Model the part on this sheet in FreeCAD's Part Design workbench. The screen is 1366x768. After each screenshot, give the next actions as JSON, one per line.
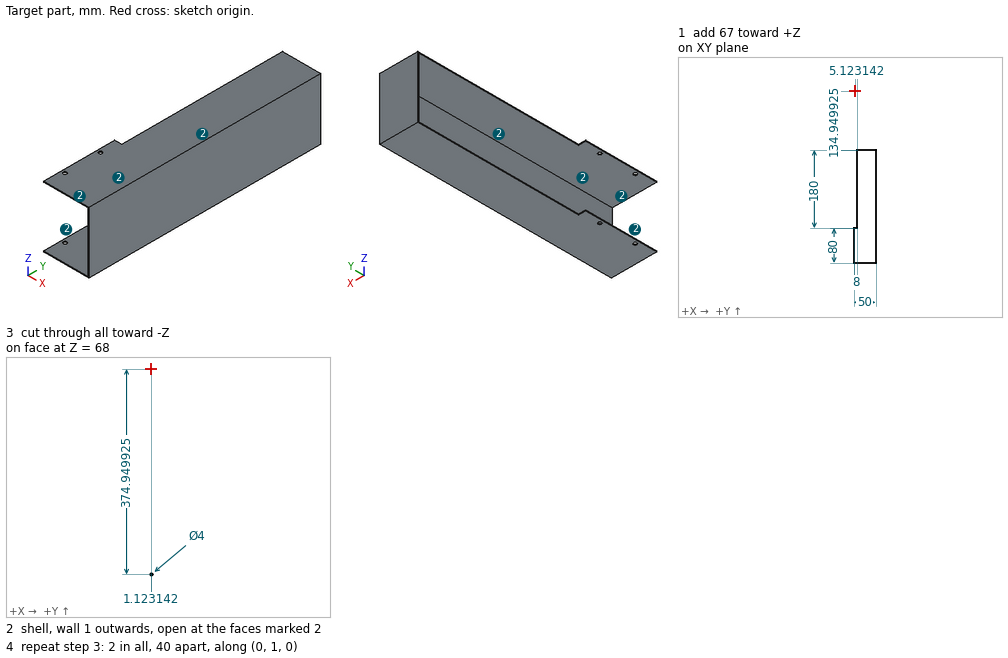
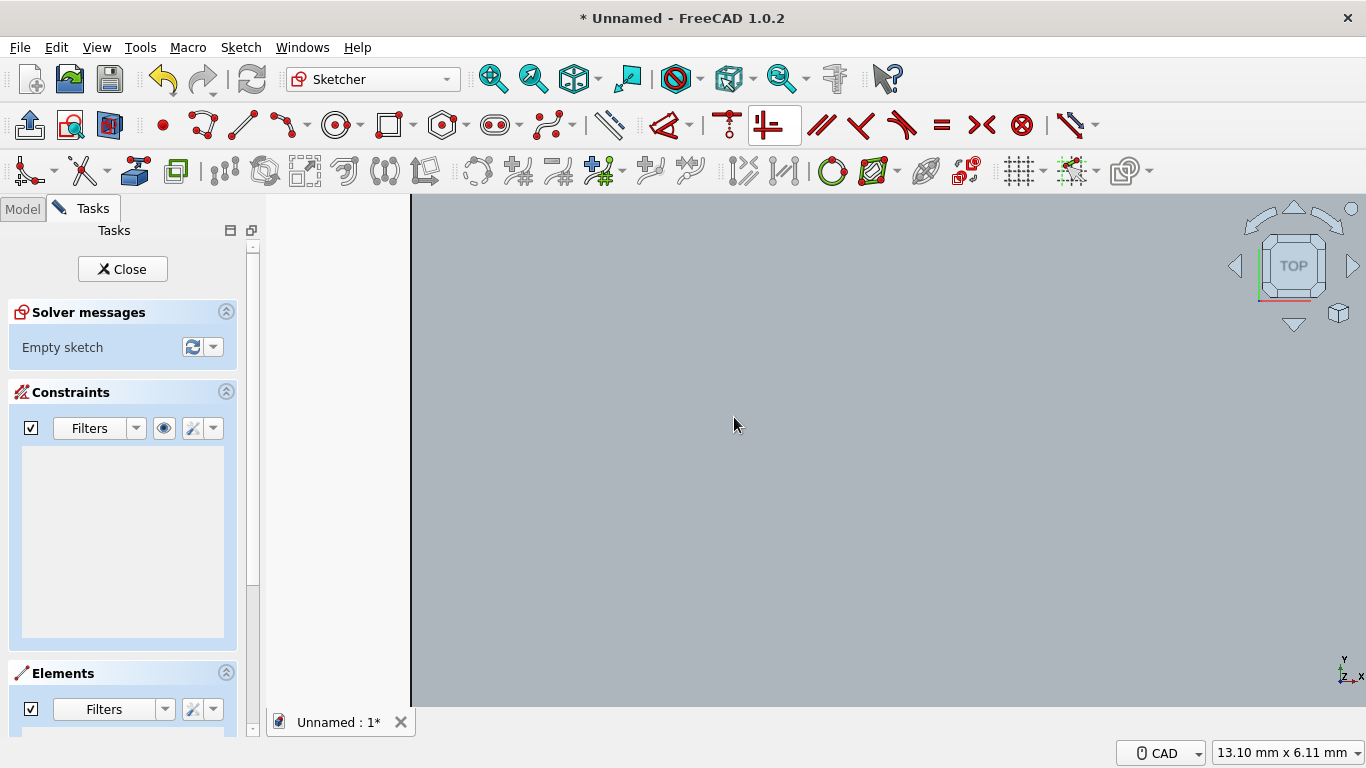
{"action": "left_click", "coordinate": [336, 126]}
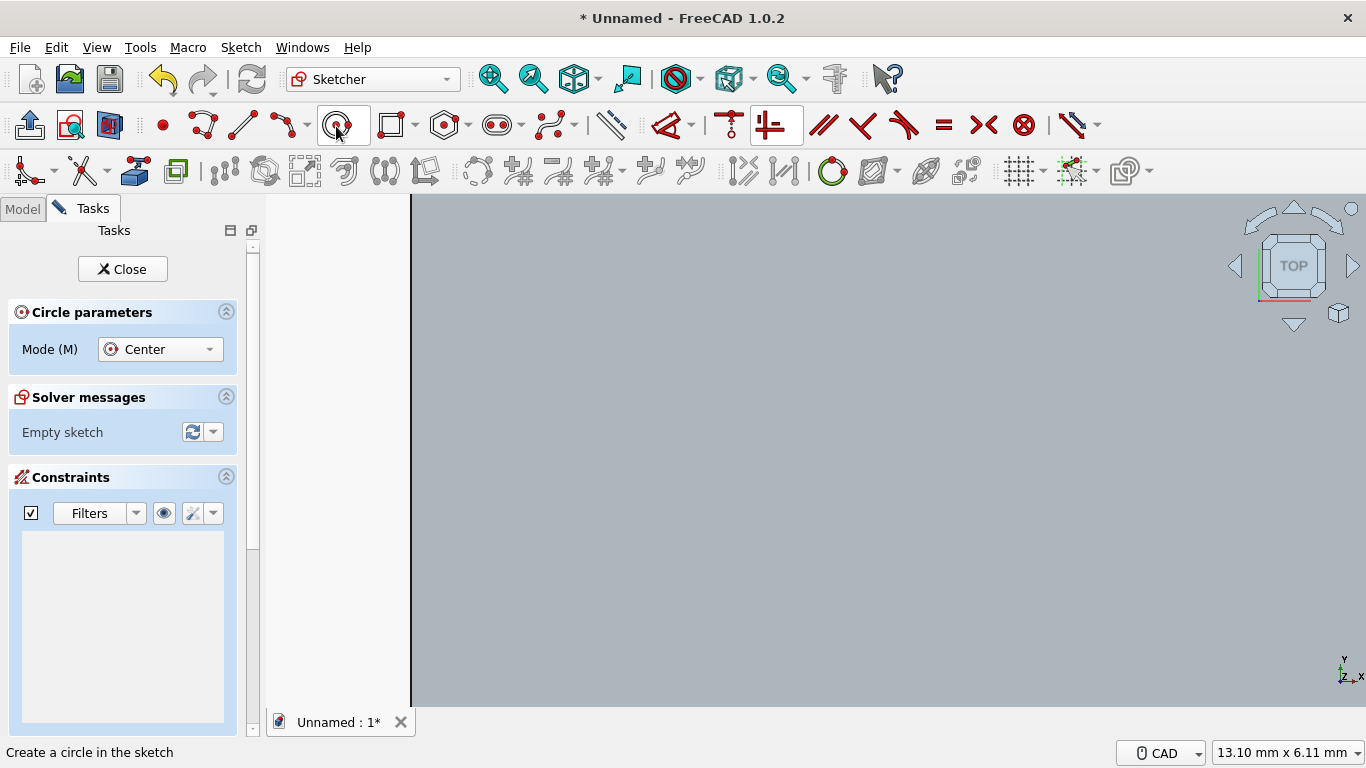
{"action": "left_click", "coordinate": [747, 449]}
{"action": "left_click", "coordinate": [866, 331]}
{"action": "key", "text": "Escape"}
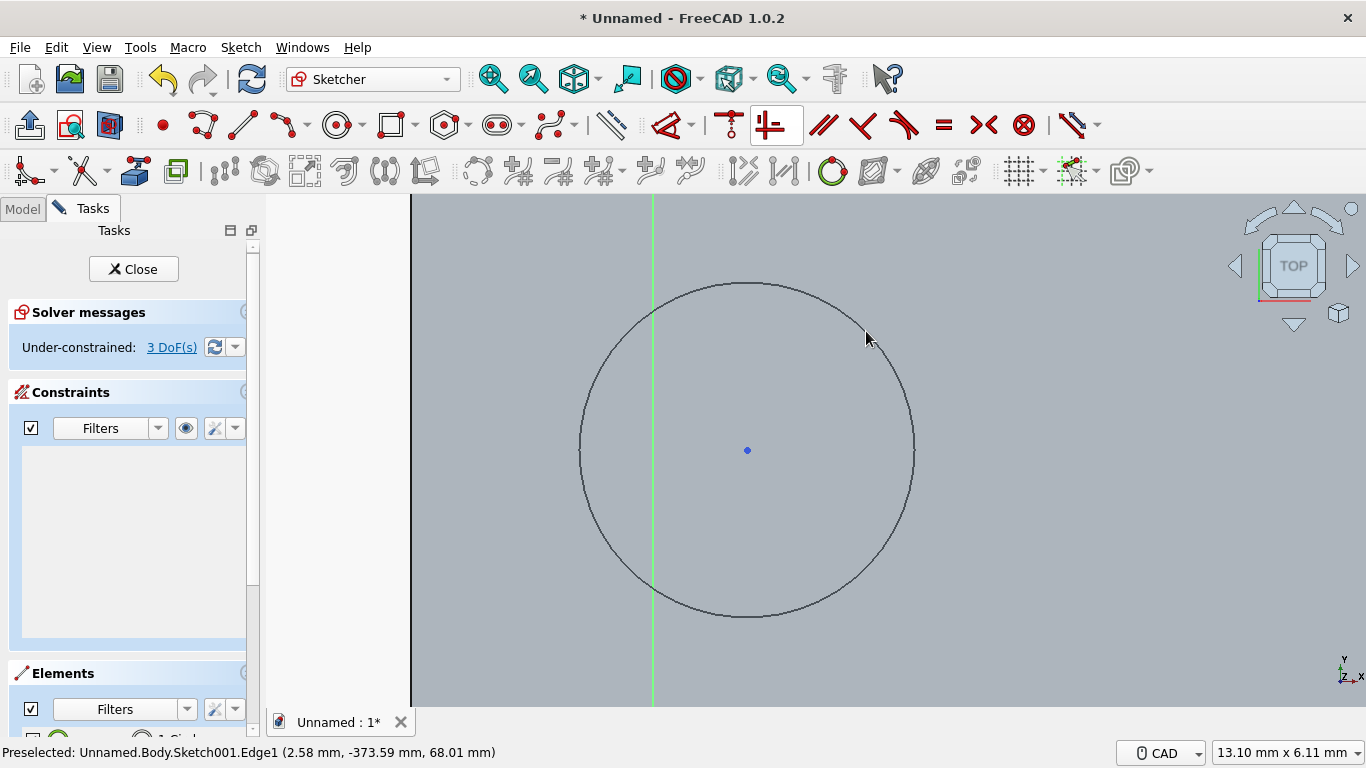
{"action": "left_click", "coordinate": [666, 126]}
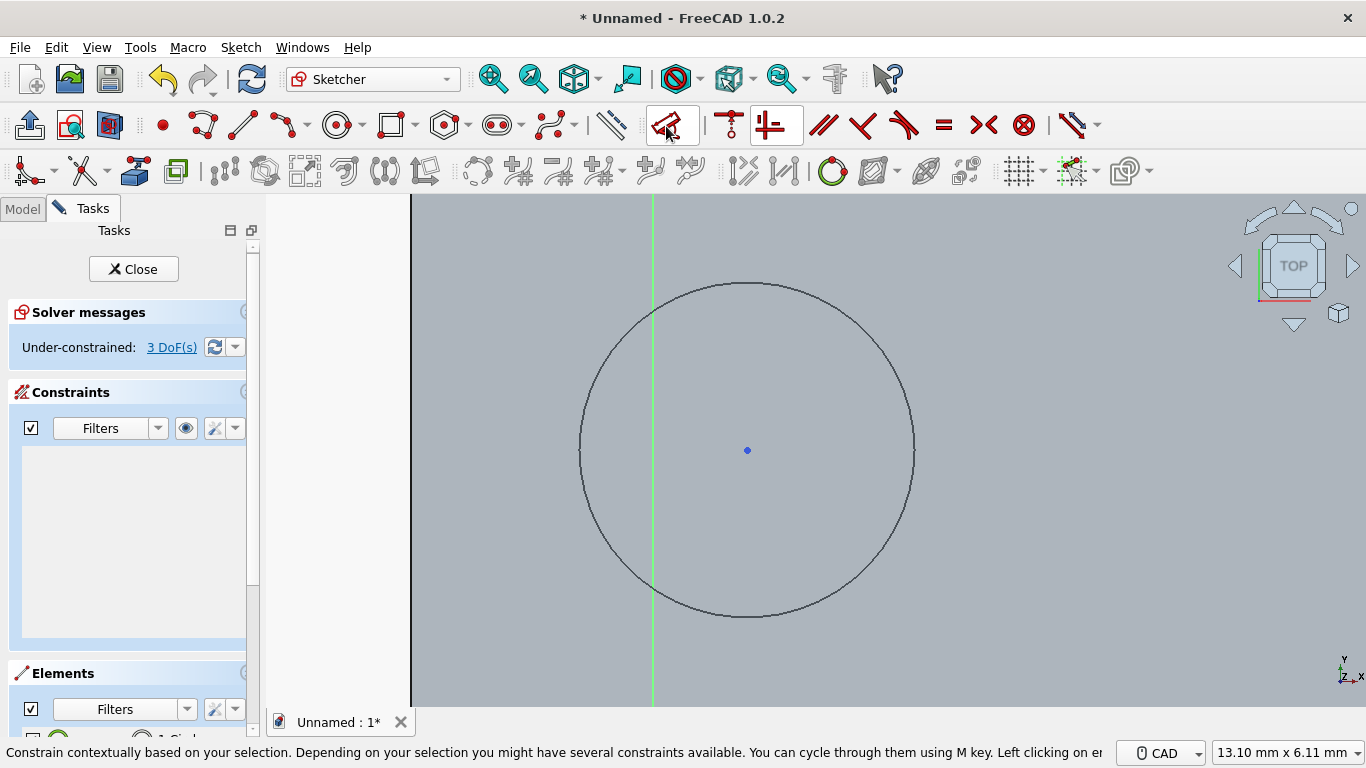
{"action": "left_click", "coordinate": [865, 331]}
{"action": "left_click", "coordinate": [888, 308]}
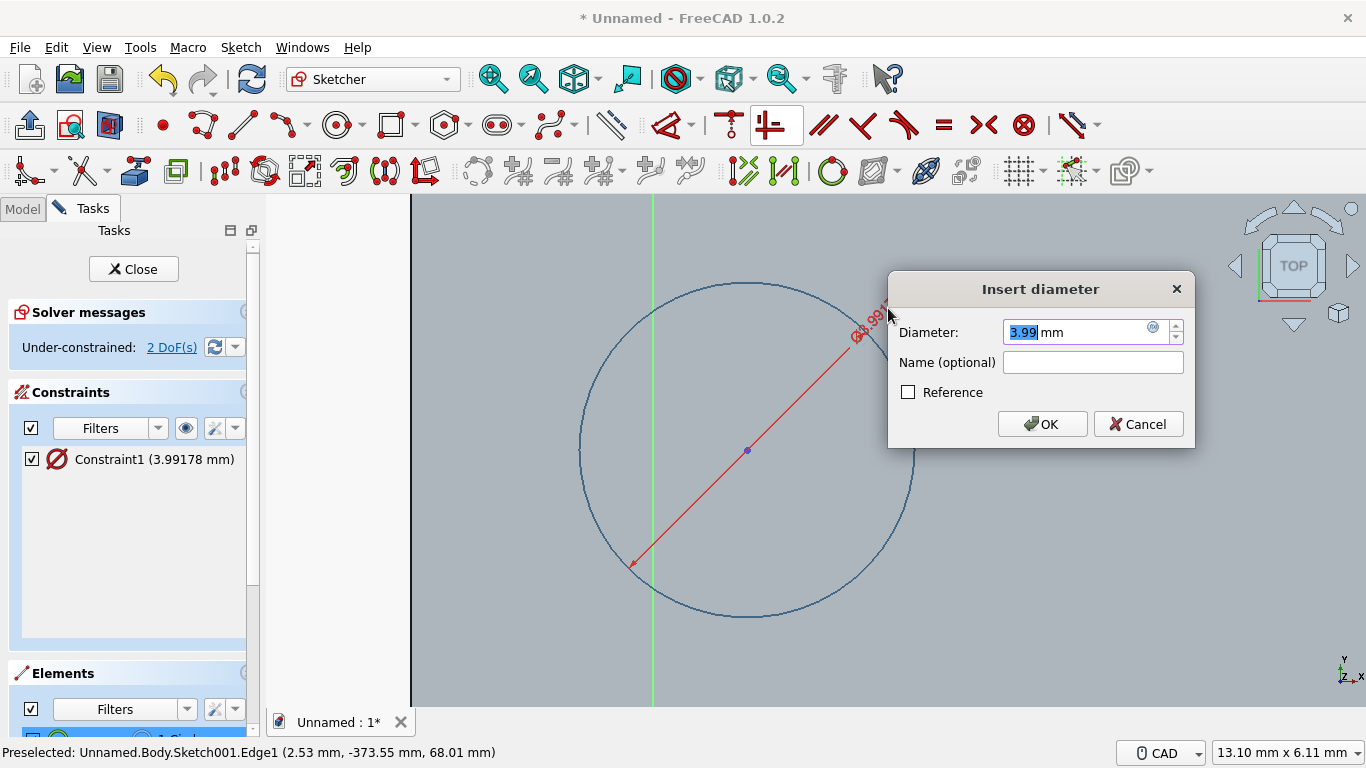
{"action": "type", "text": "4"}
{"action": "key", "text": "Return"}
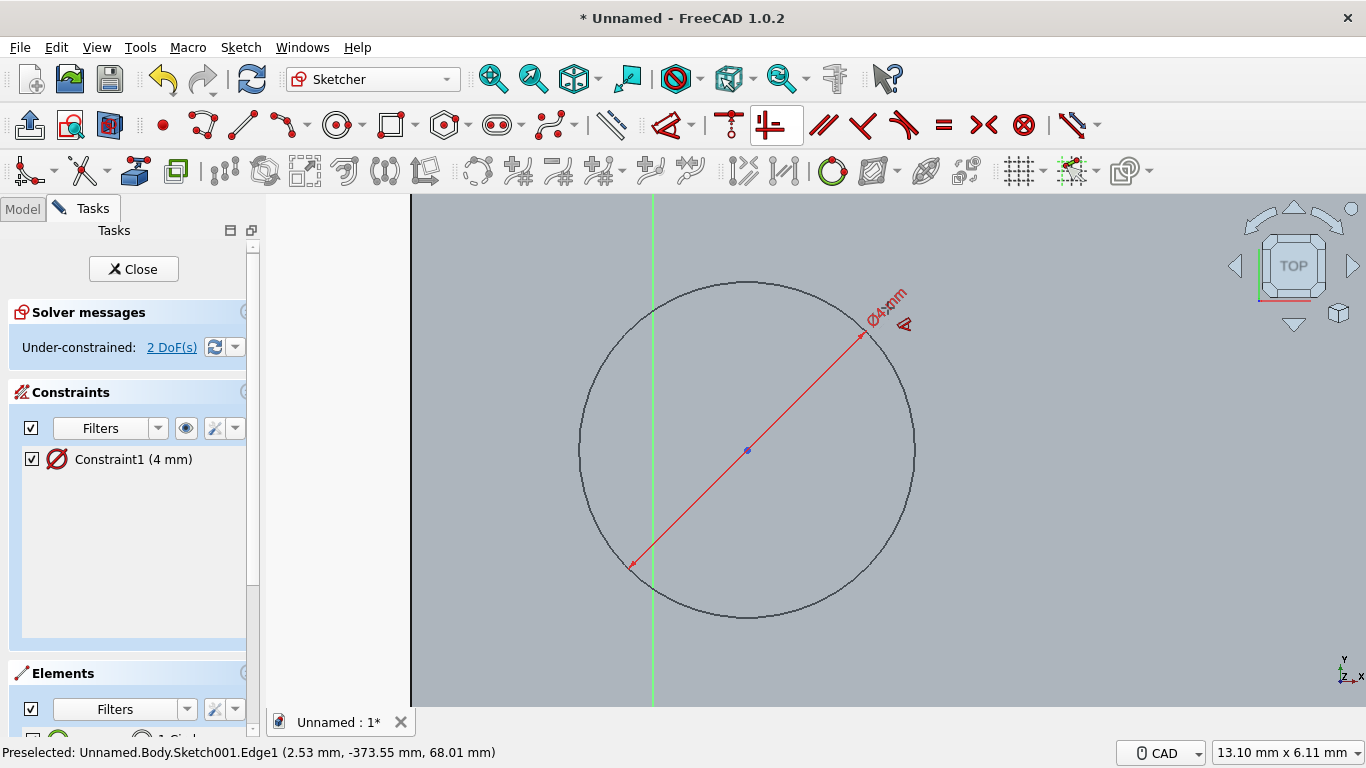
{"action": "left_click", "coordinate": [747, 450]}
{"action": "left_click", "coordinate": [700, 484]}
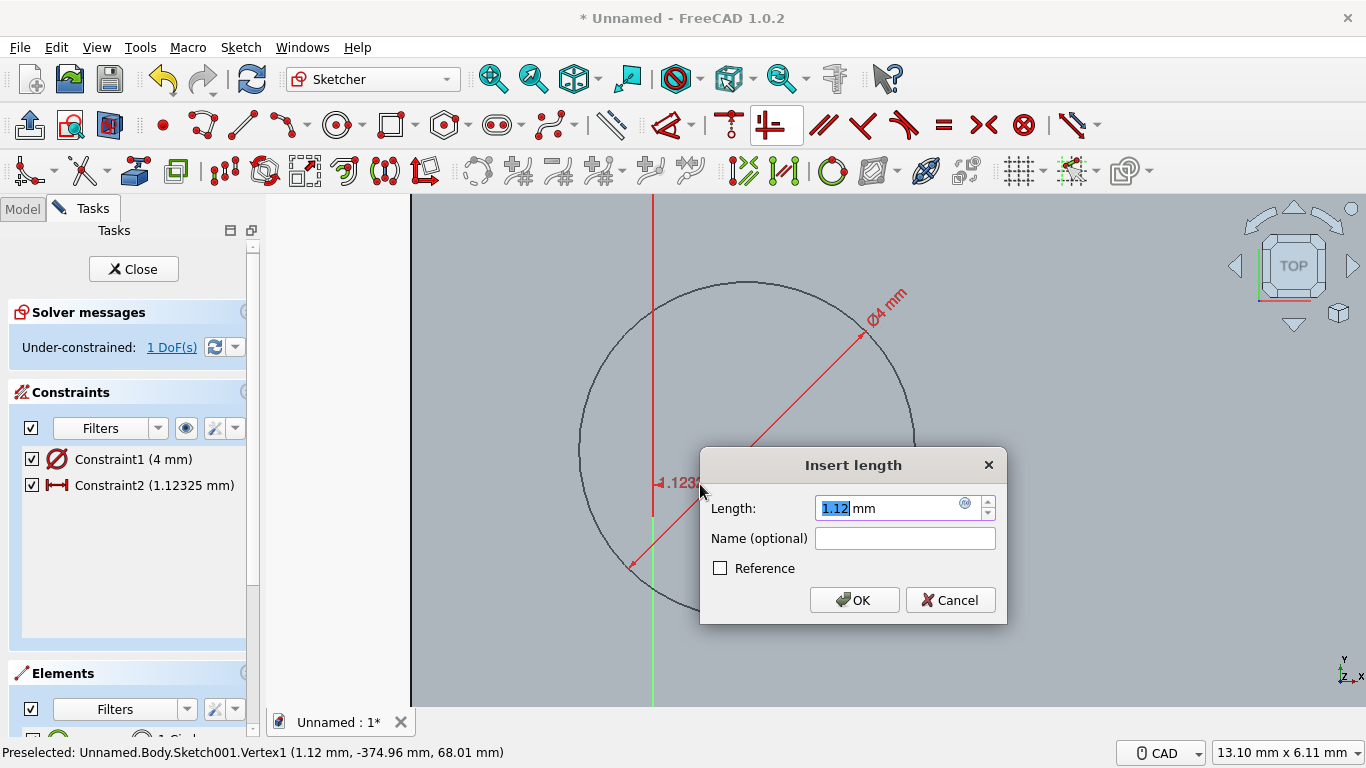
{"action": "type", "text": "1.123142"}
{"action": "key", "text": "Return"}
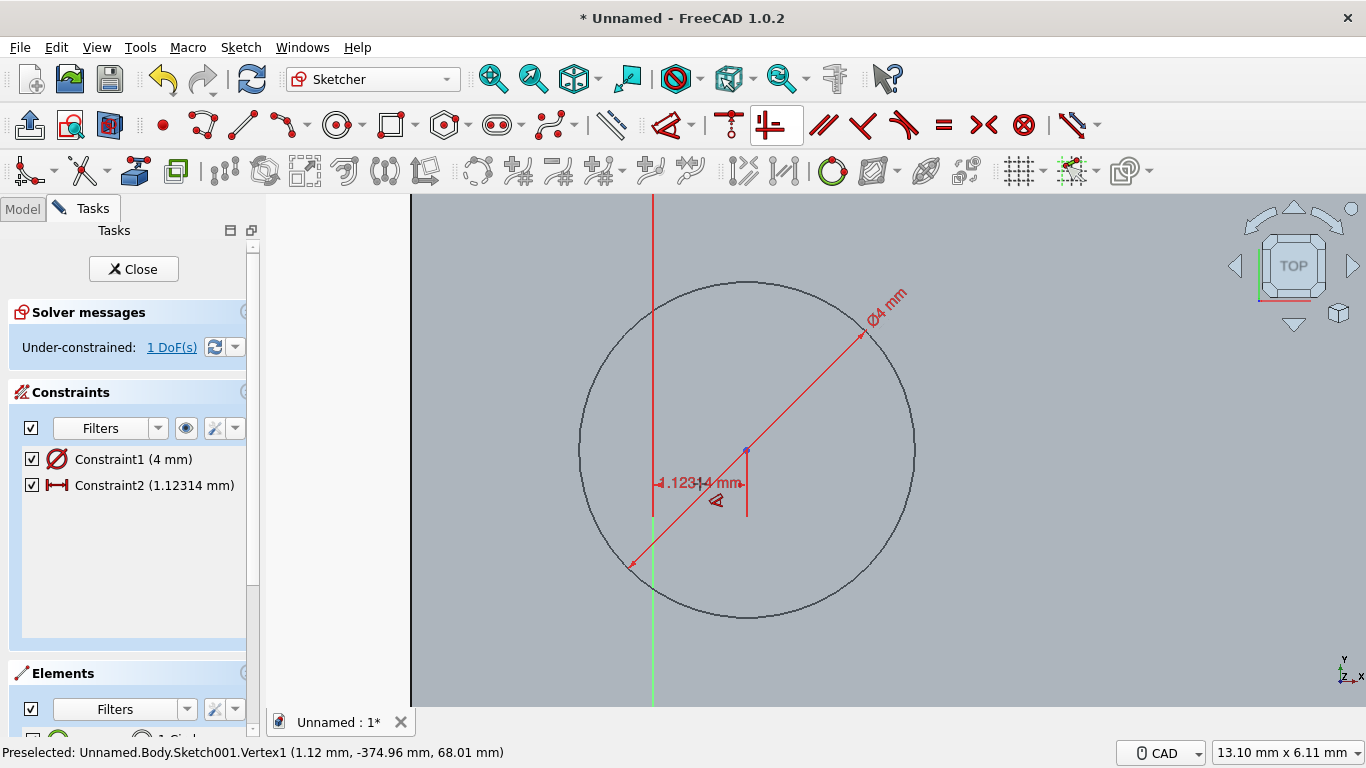
{"action": "left_click", "coordinate": [747, 450]}
{"action": "left_click", "coordinate": [619, 284]}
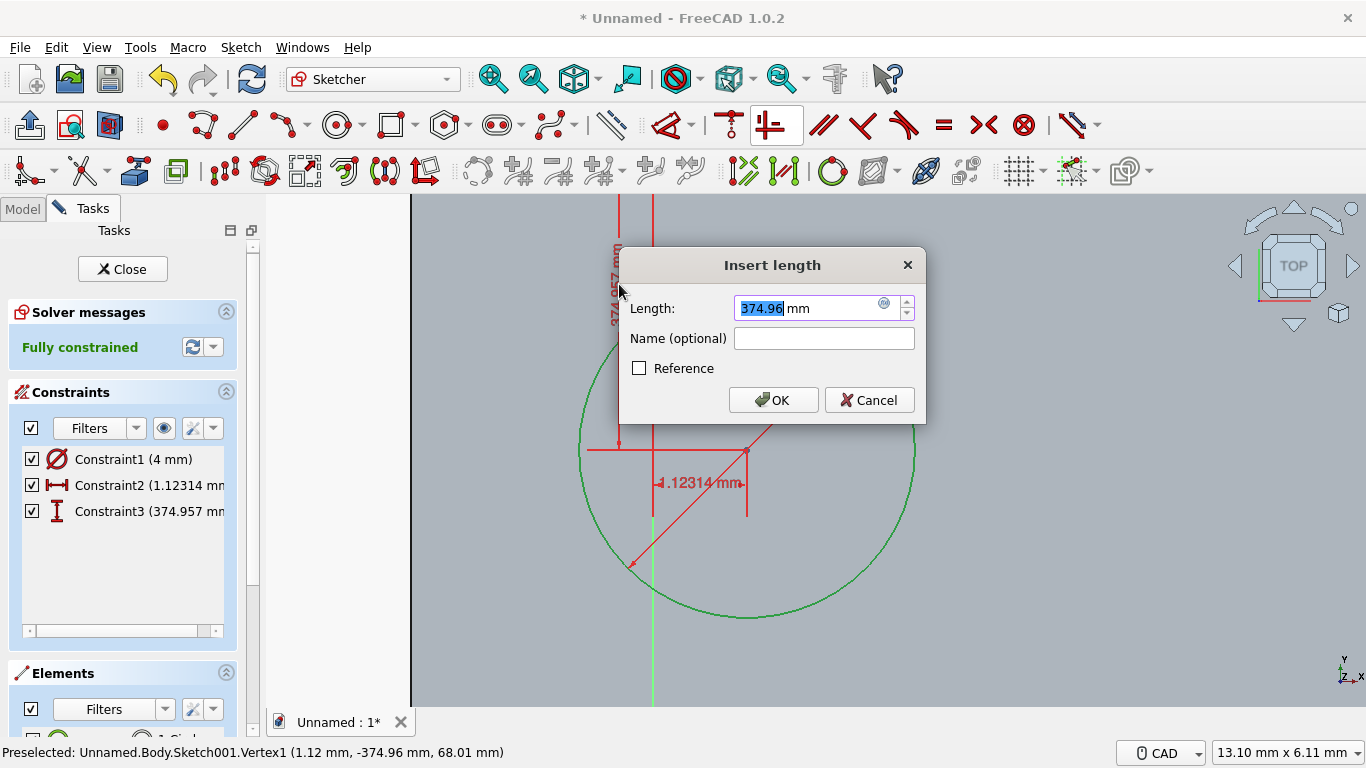
{"action": "type", "text": "374.949925"}
{"action": "key", "text": "Return"}
{"action": "key", "text": "Escape"}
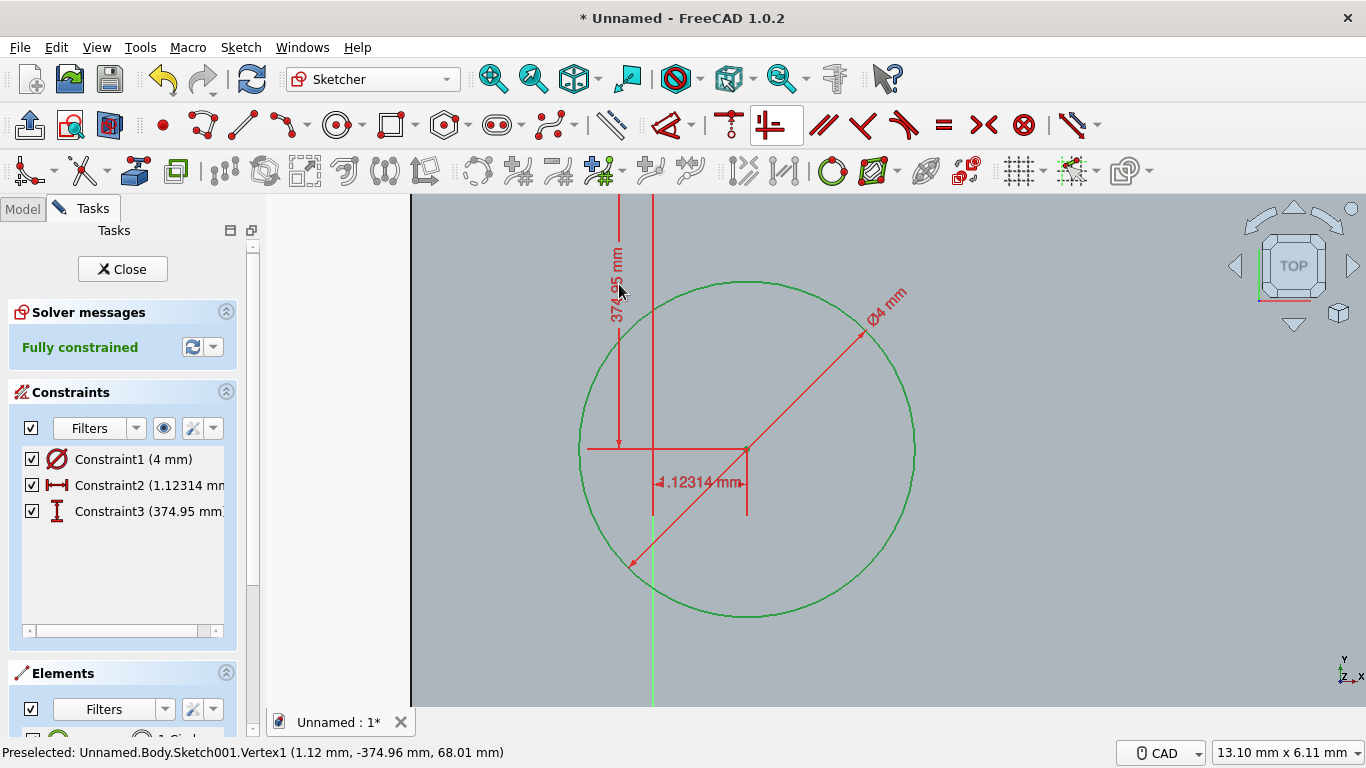
{"action": "left_click", "coordinate": [123, 269]}